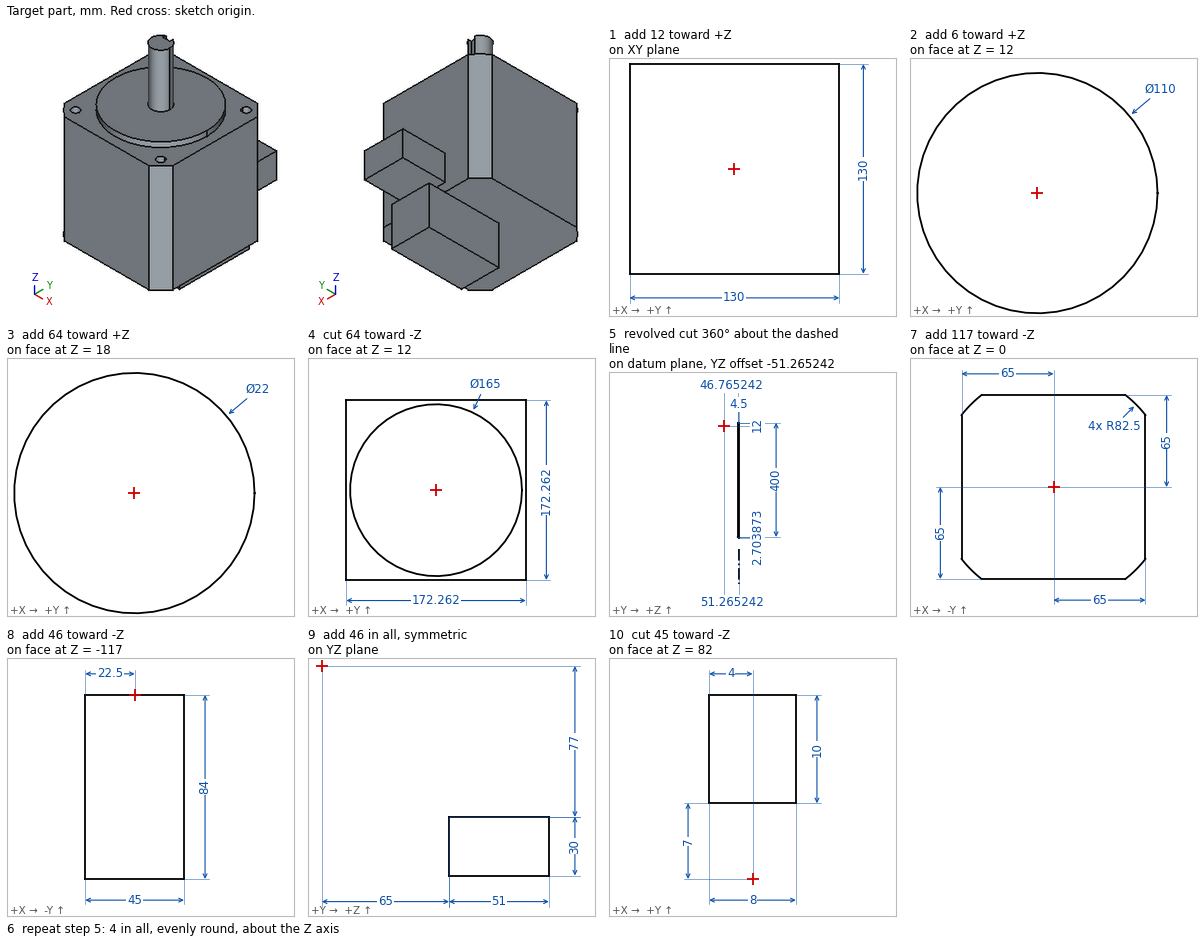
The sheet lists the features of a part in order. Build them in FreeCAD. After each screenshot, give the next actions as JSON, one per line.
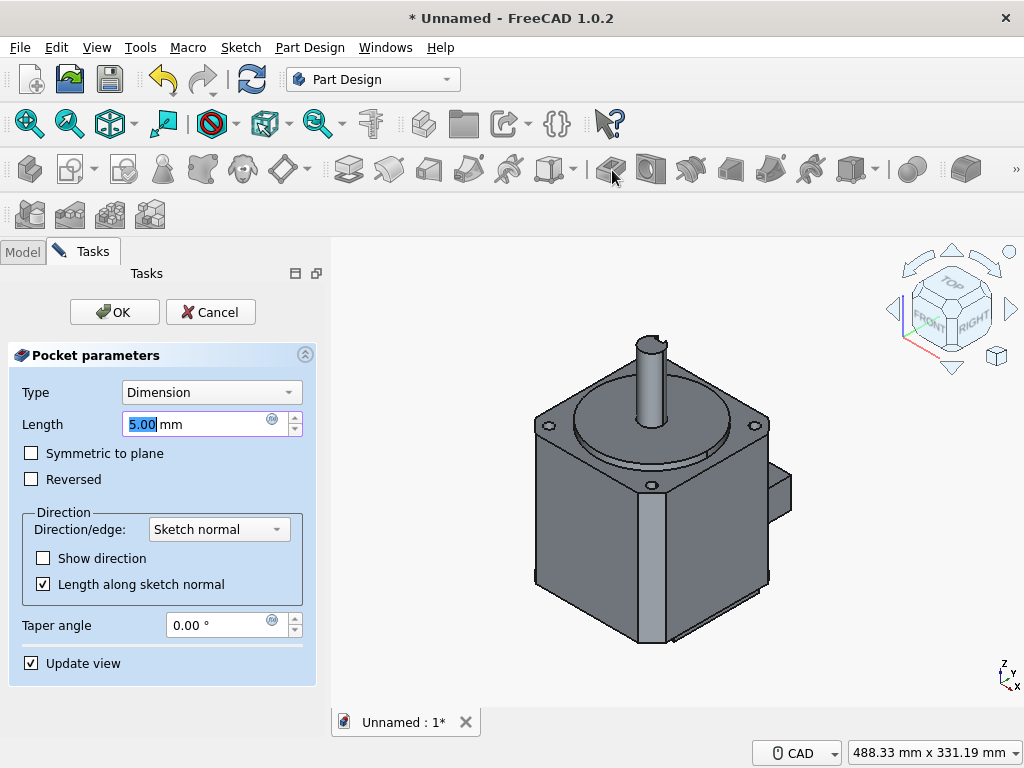
{"action": "type", "text": "45"}
{"action": "key", "text": "Tab"}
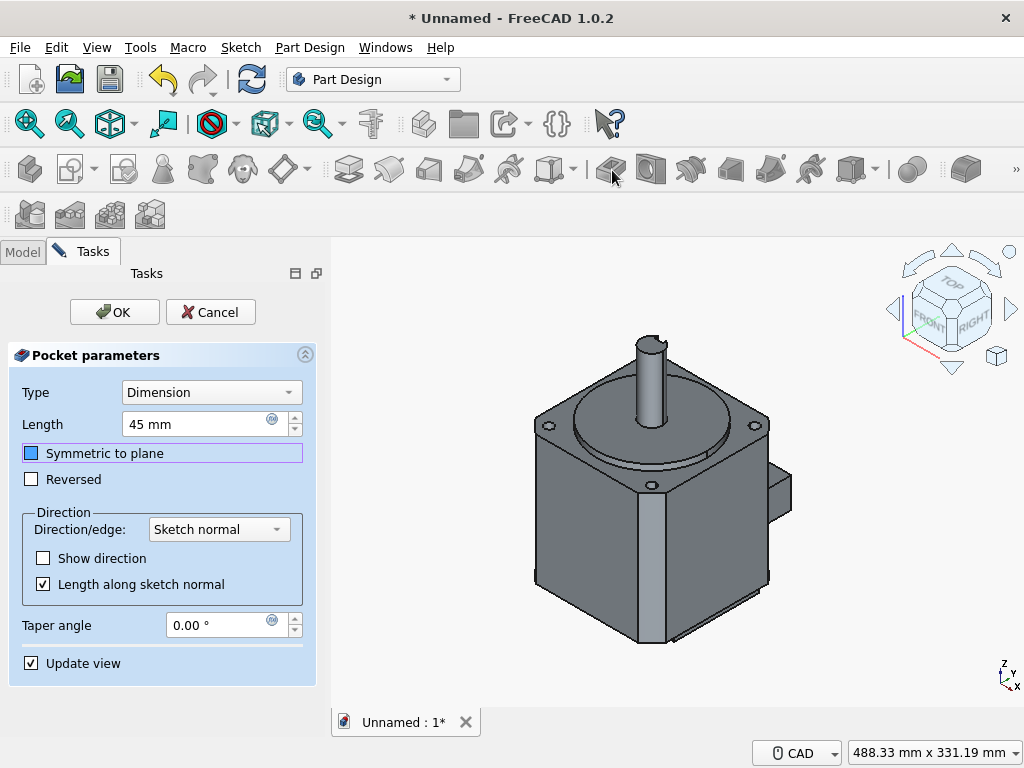
{"action": "left_click", "coordinate": [115, 312]}